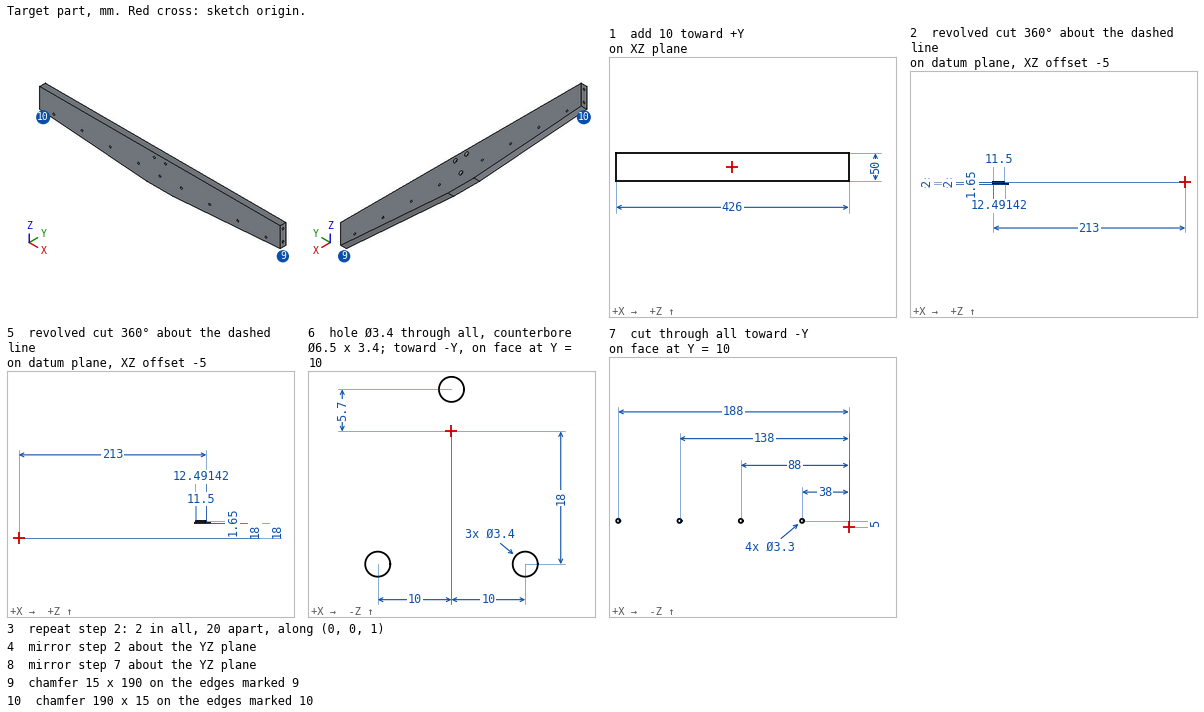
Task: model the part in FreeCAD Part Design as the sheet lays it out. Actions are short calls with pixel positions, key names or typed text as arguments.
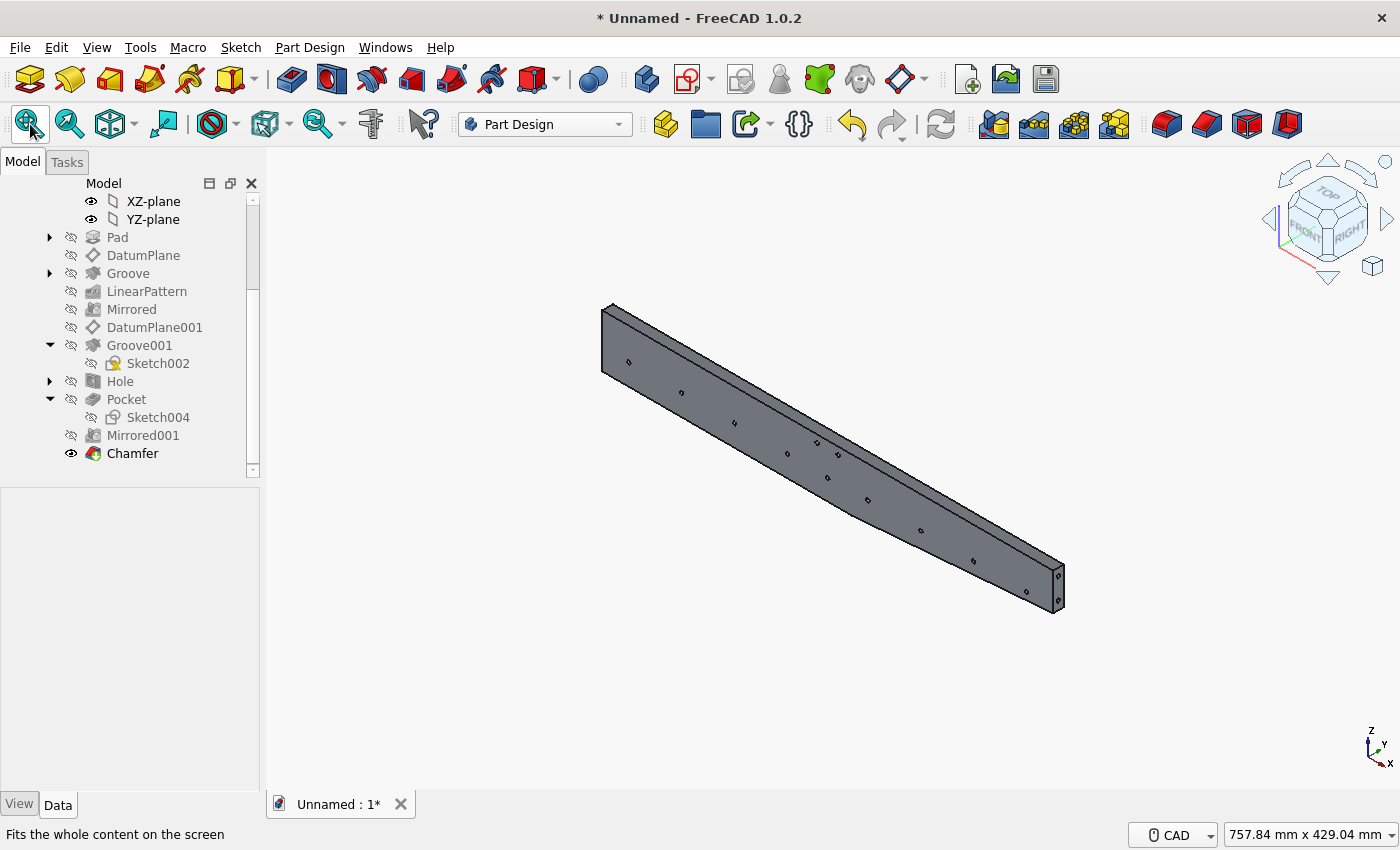
scroll(608, 367, up, 5)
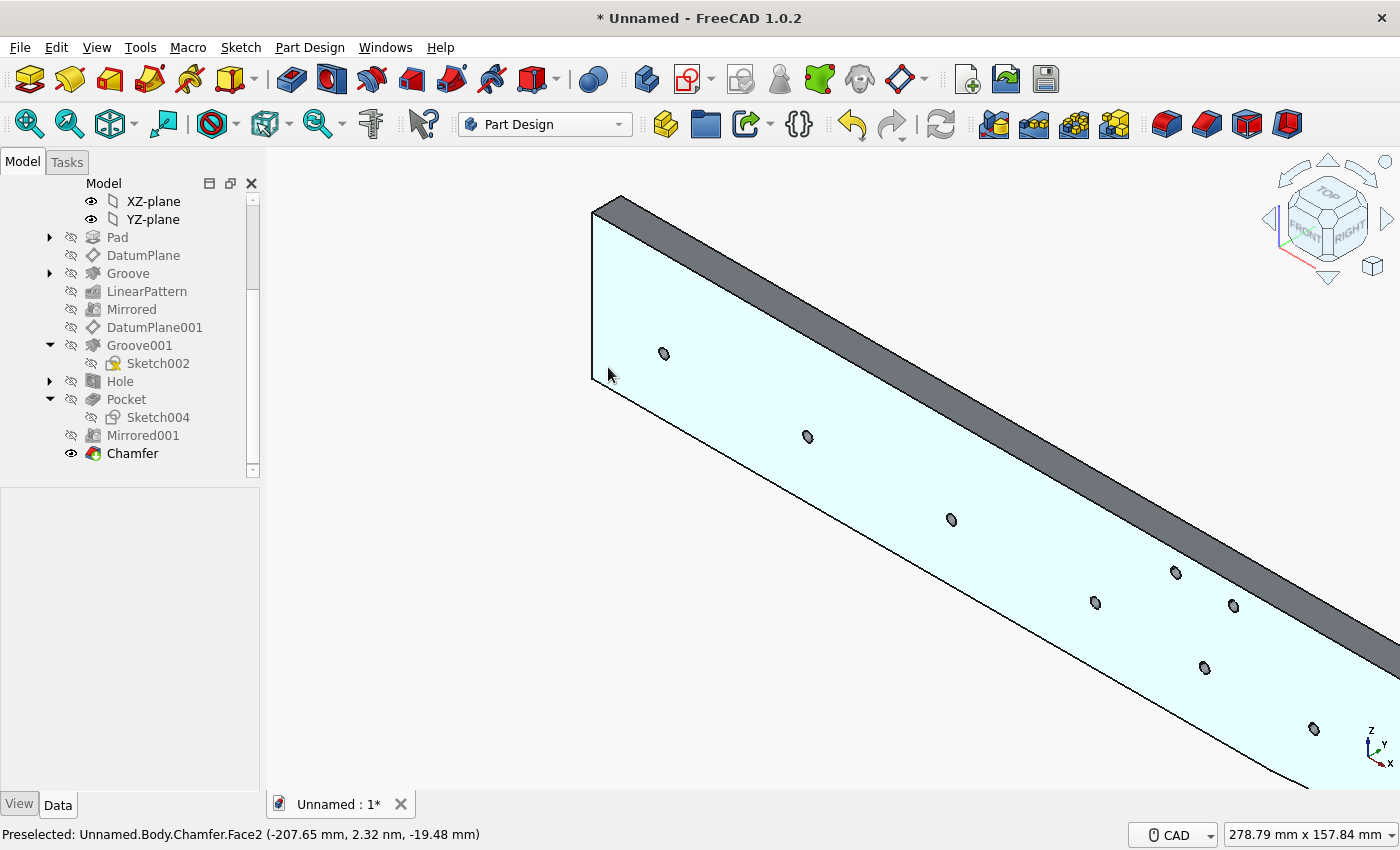
click(30, 124)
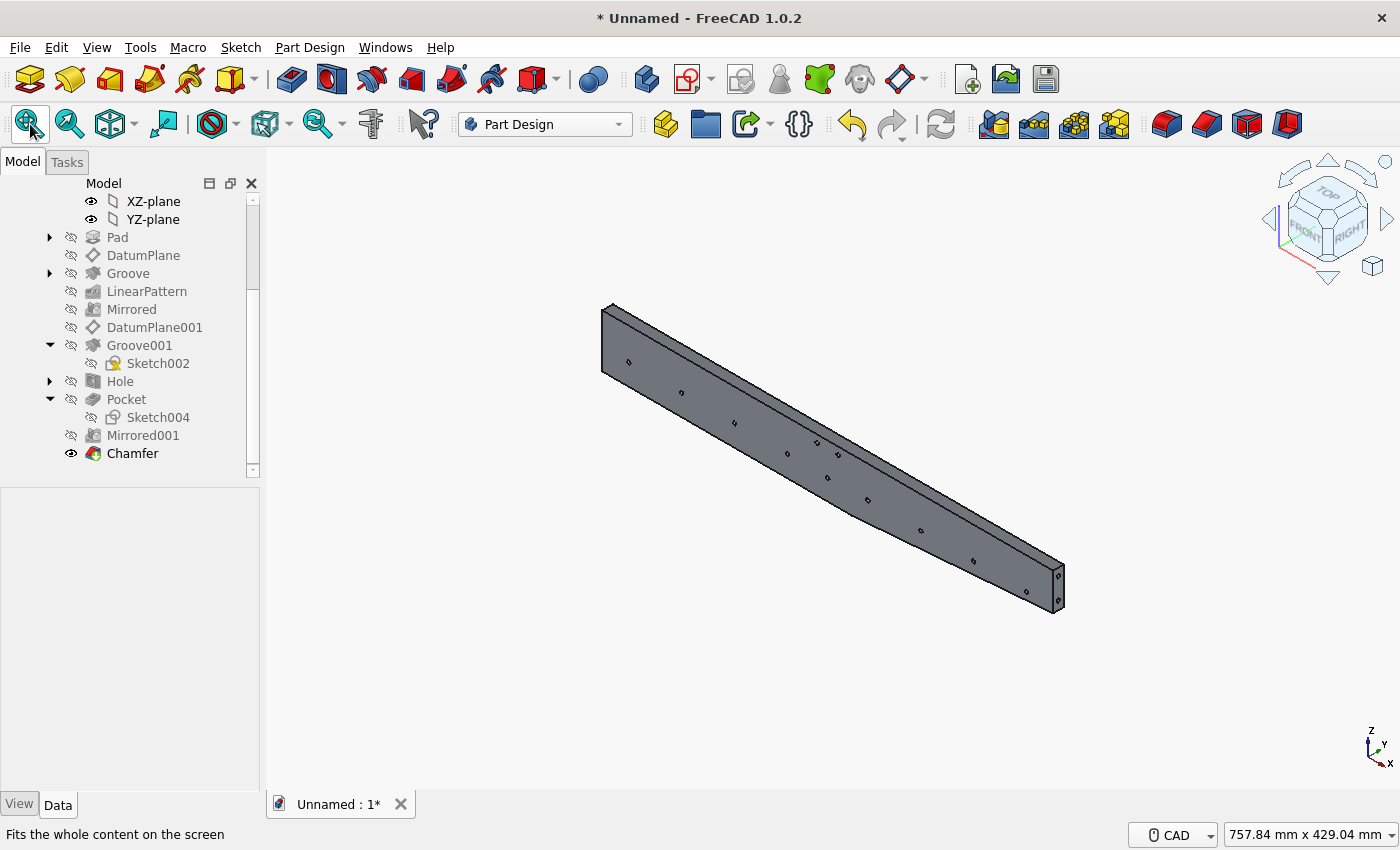
key(2)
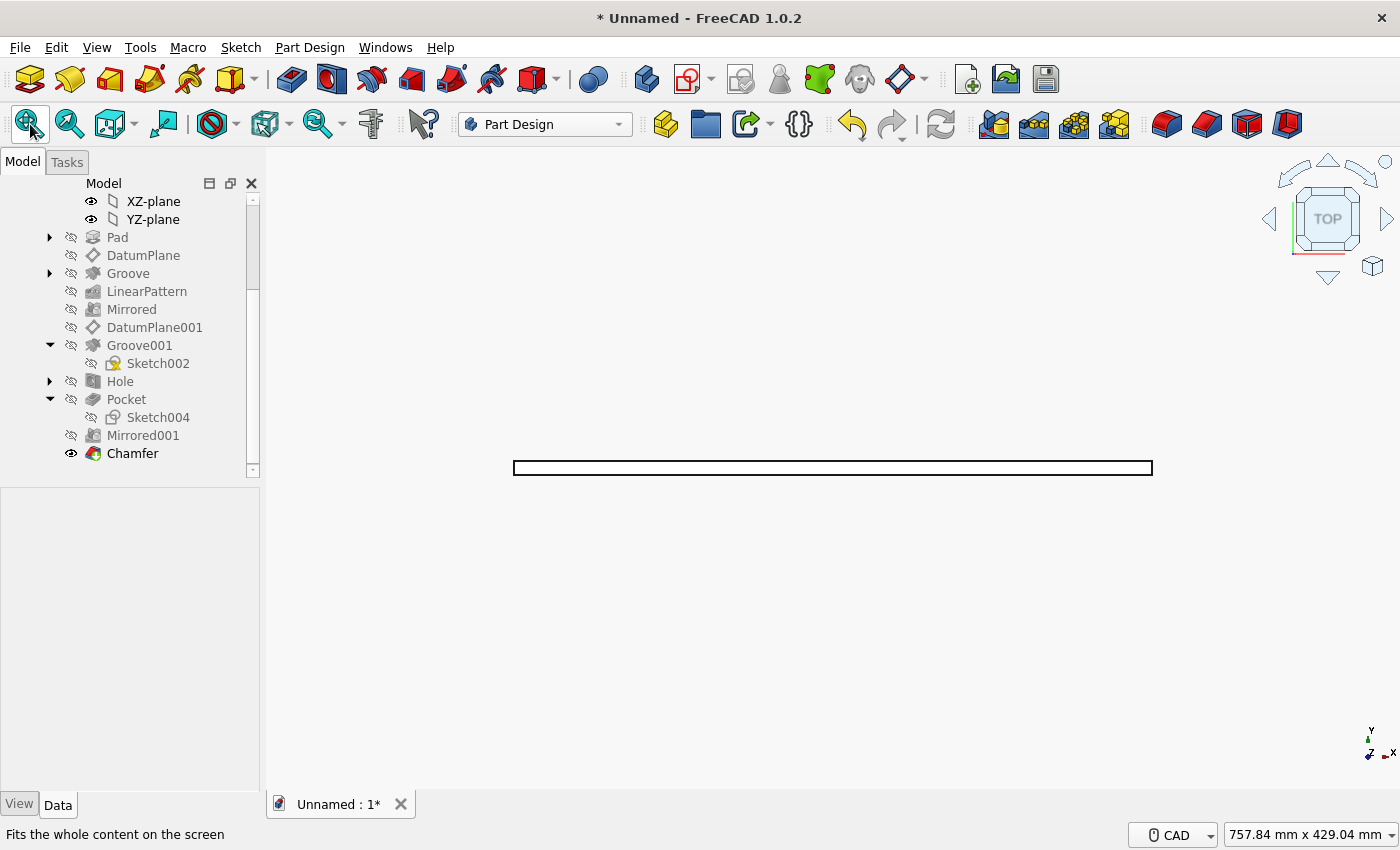
scroll(514, 467, up, 5)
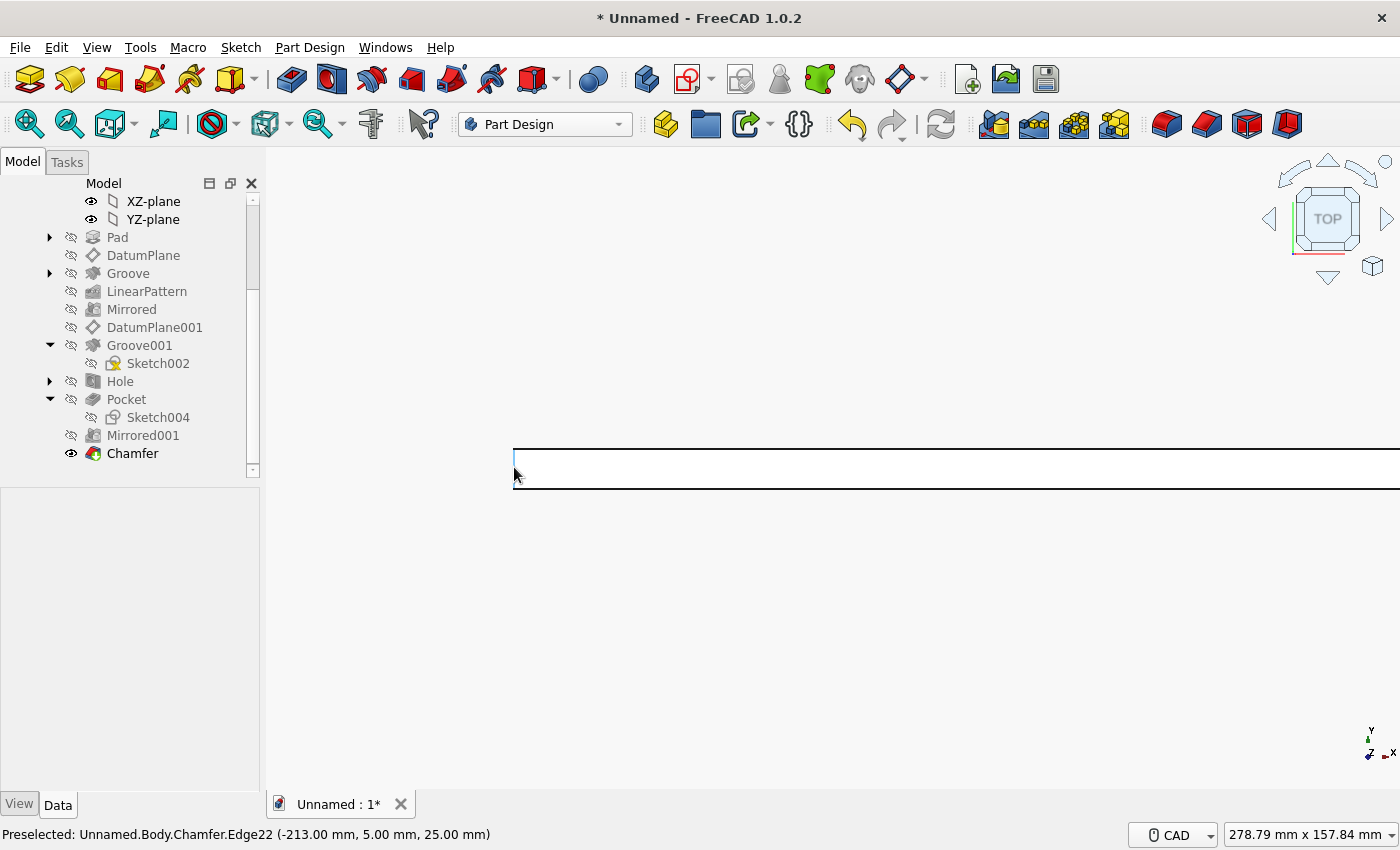
click(30, 124)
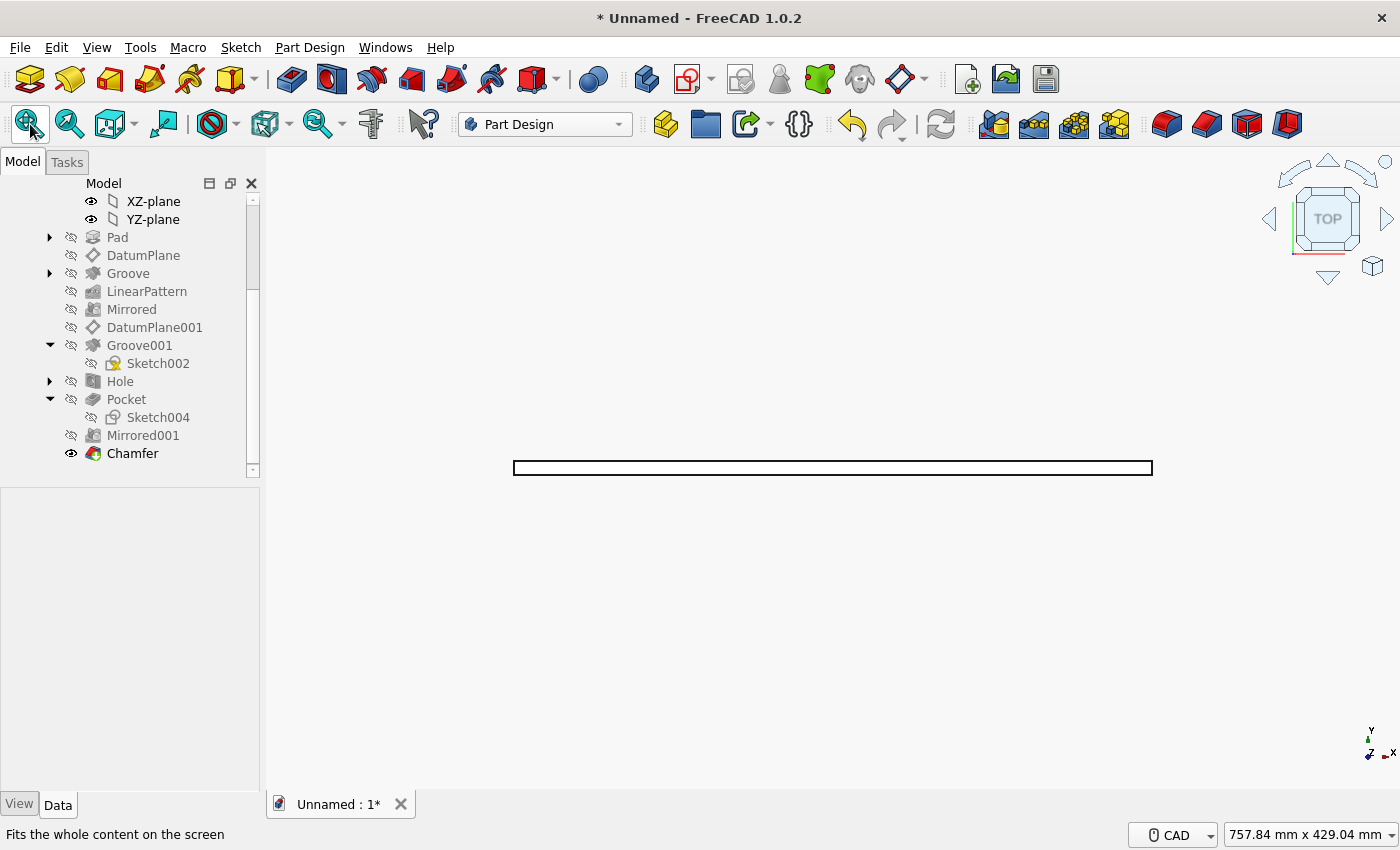
key(1)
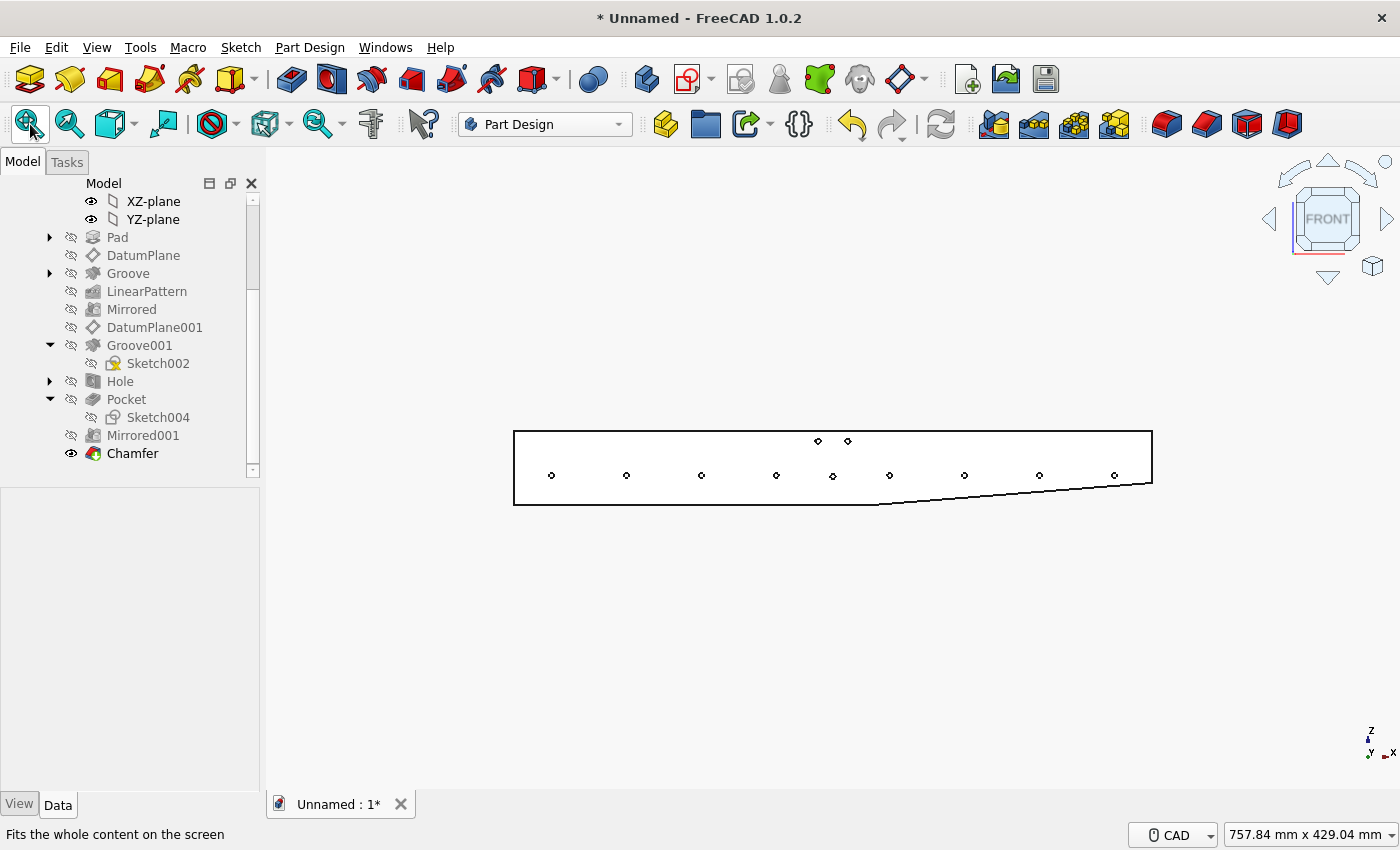
scroll(514, 504, up, 5)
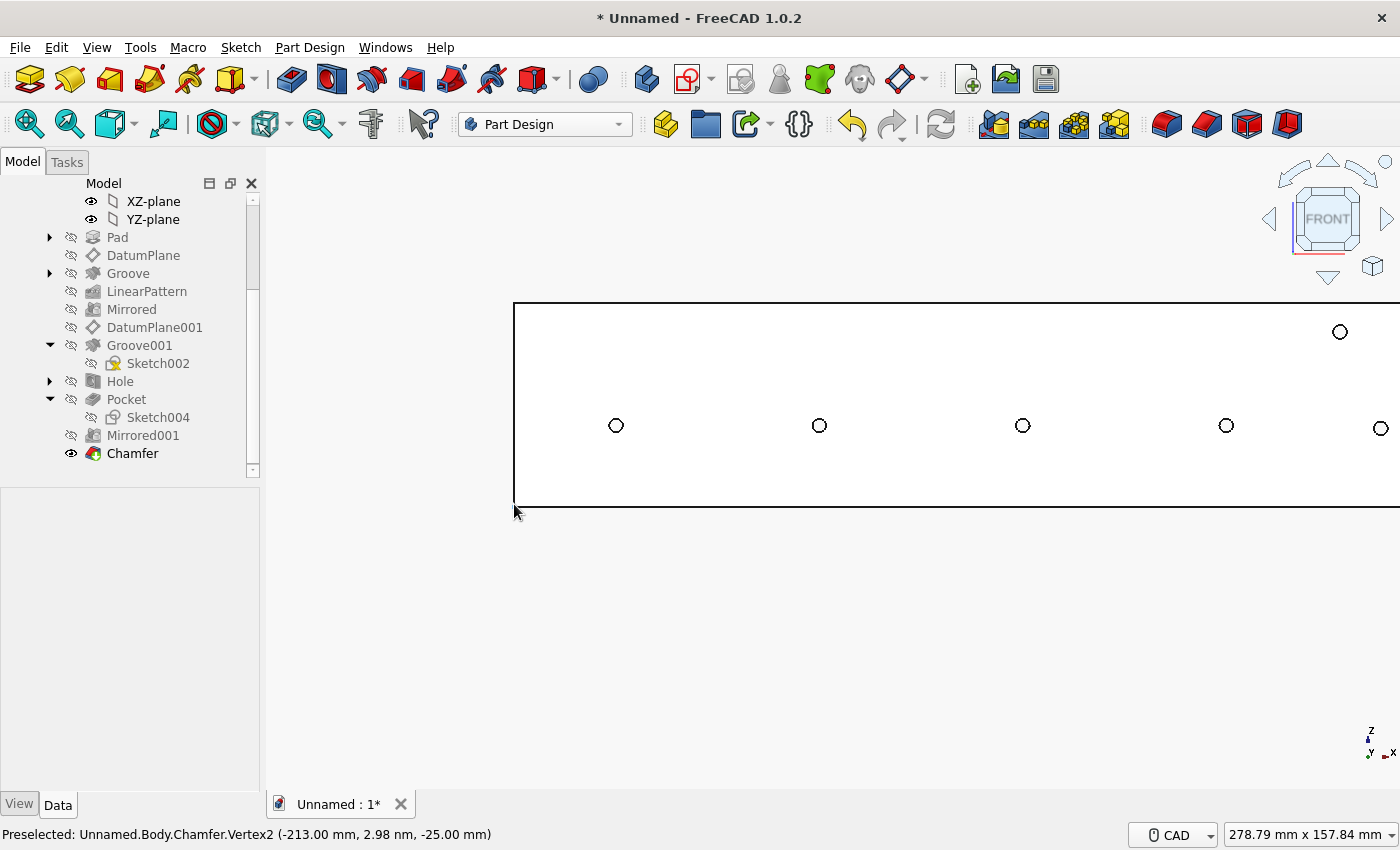
key(v)
key(f)